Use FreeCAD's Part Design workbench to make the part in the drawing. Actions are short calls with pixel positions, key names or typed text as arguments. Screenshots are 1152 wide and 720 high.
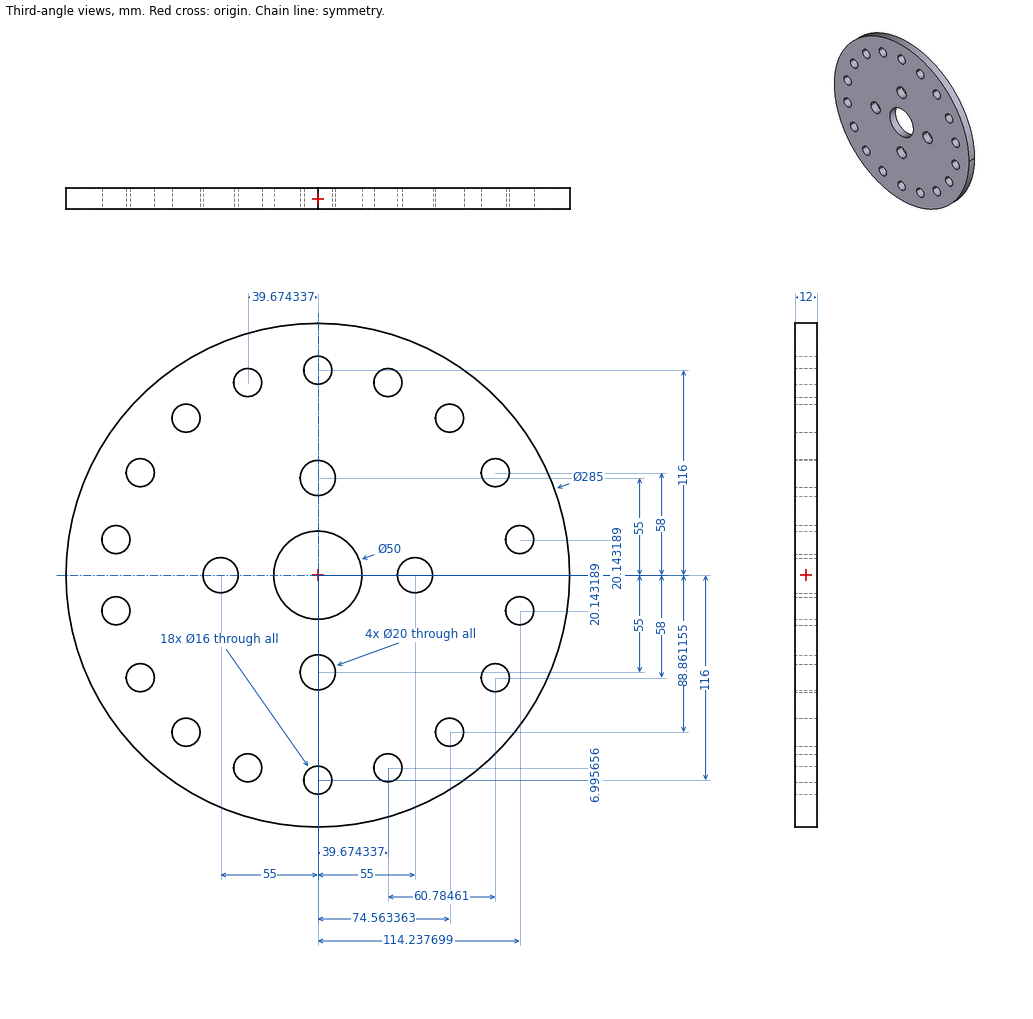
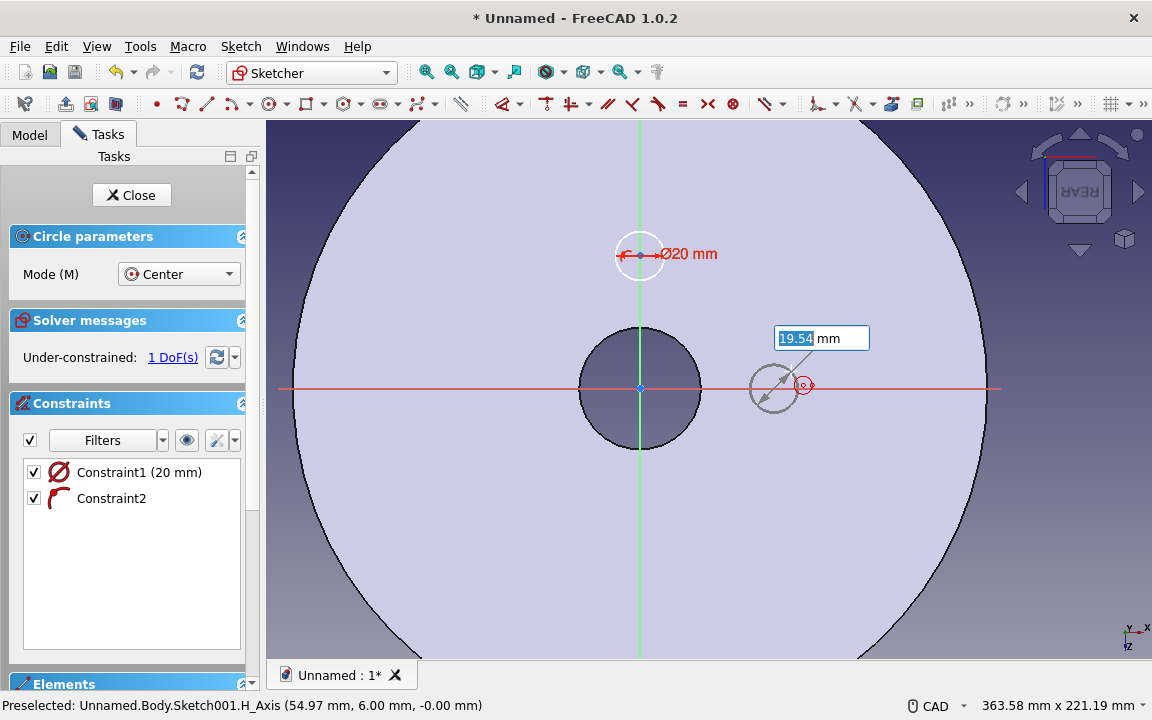
text(20)
key(Return)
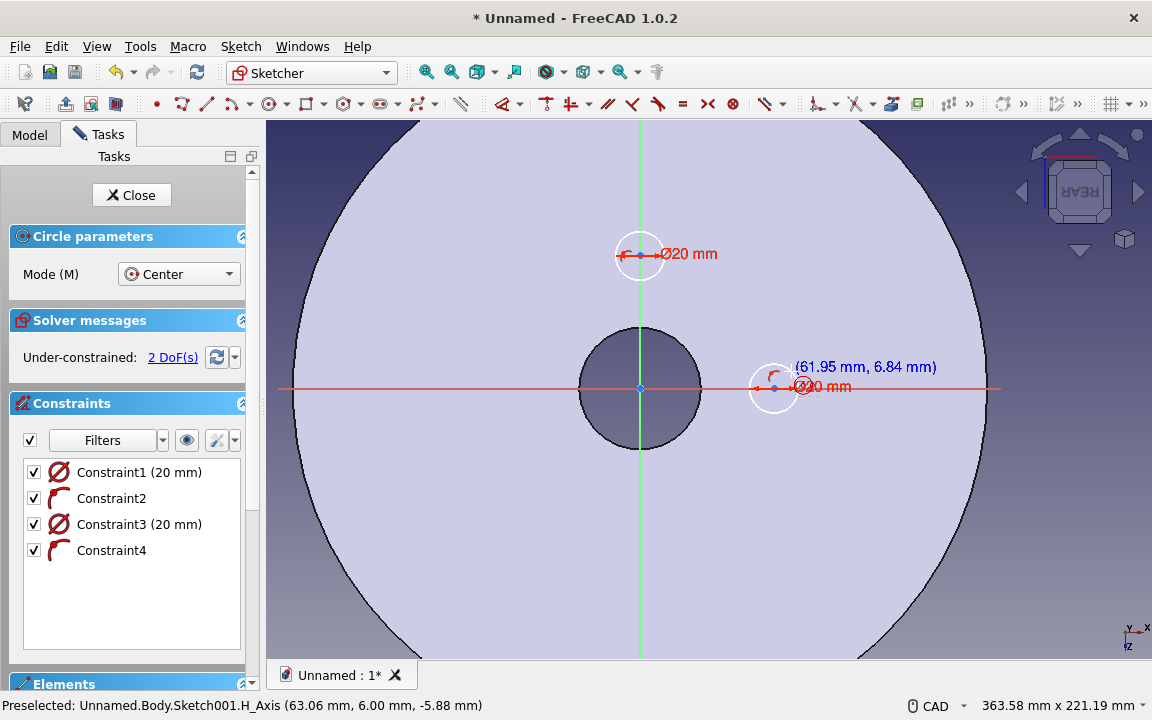
click(640, 523)
move(657, 505)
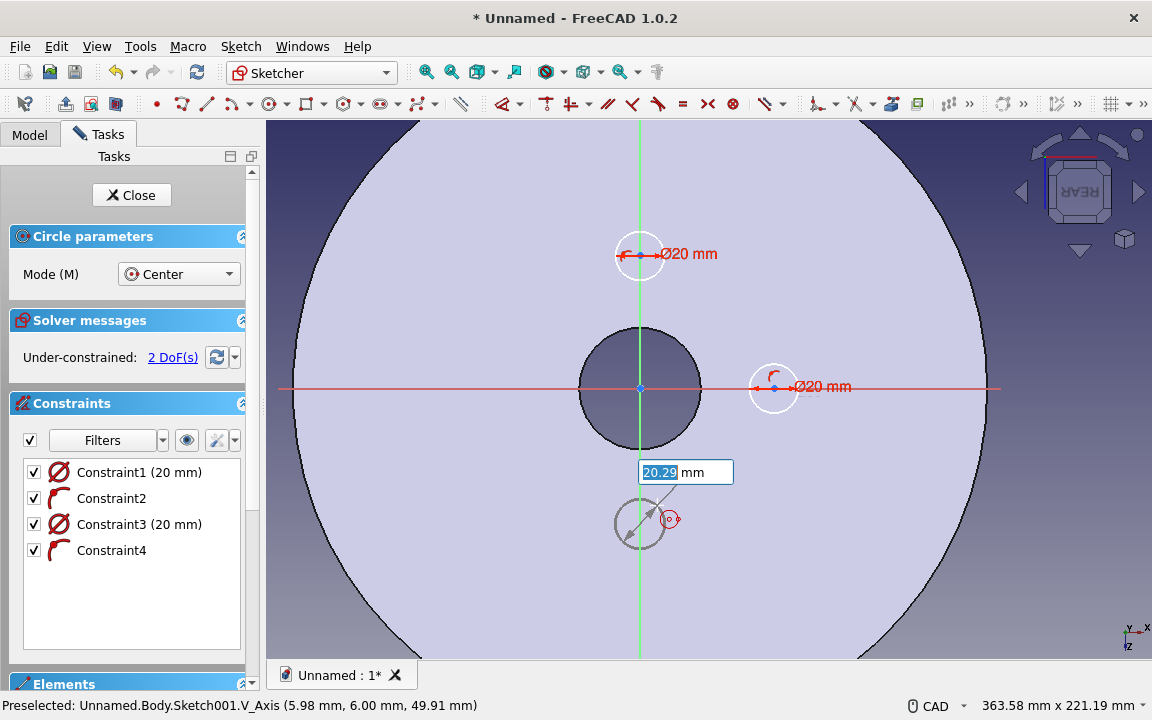
text(20)
key(Return)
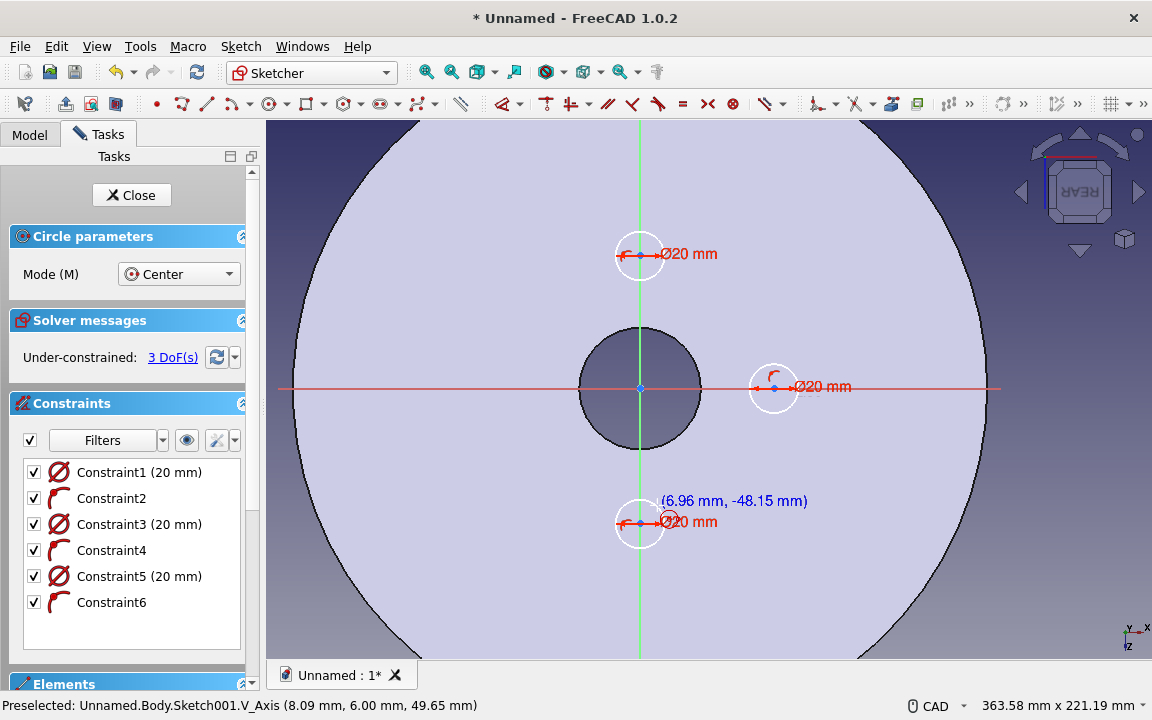
click(506, 389)
move(523, 371)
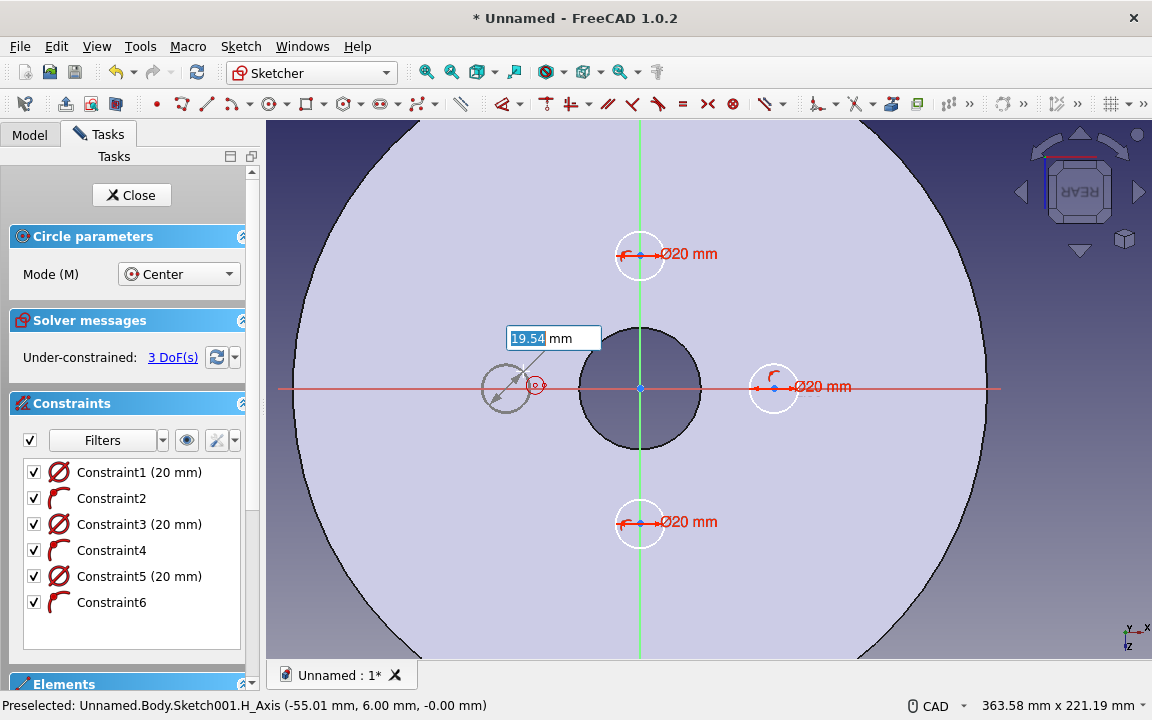
text(20)
key(Return)
key(Escape)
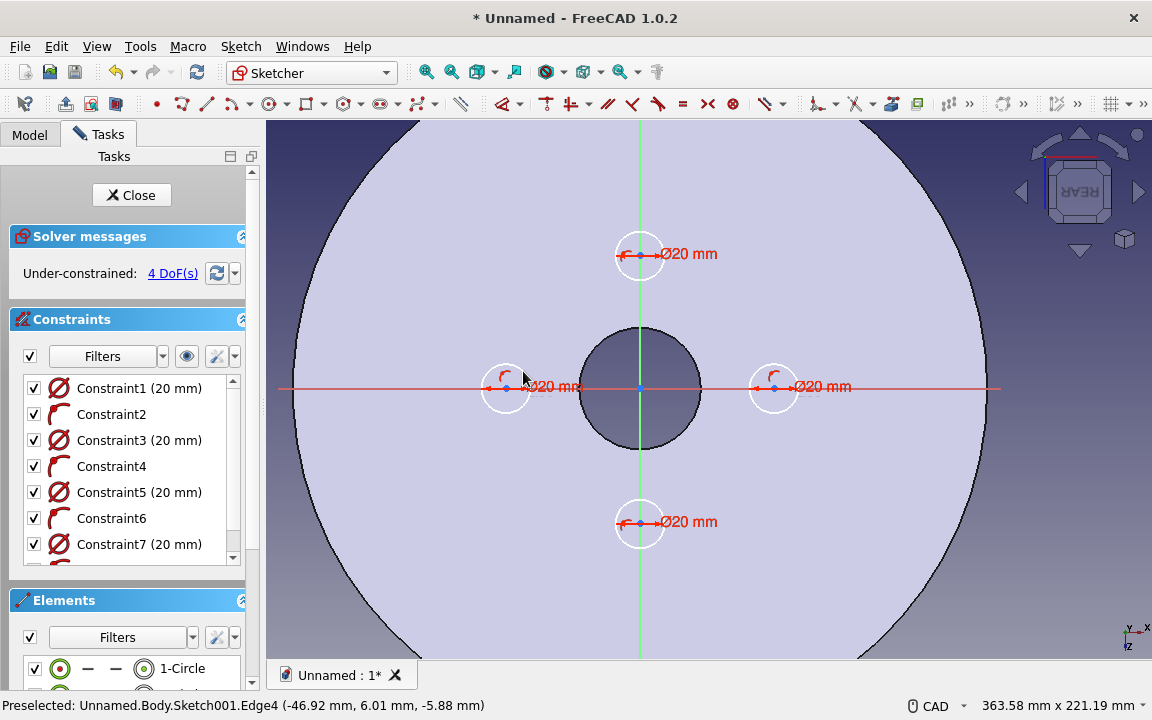
click(502, 104)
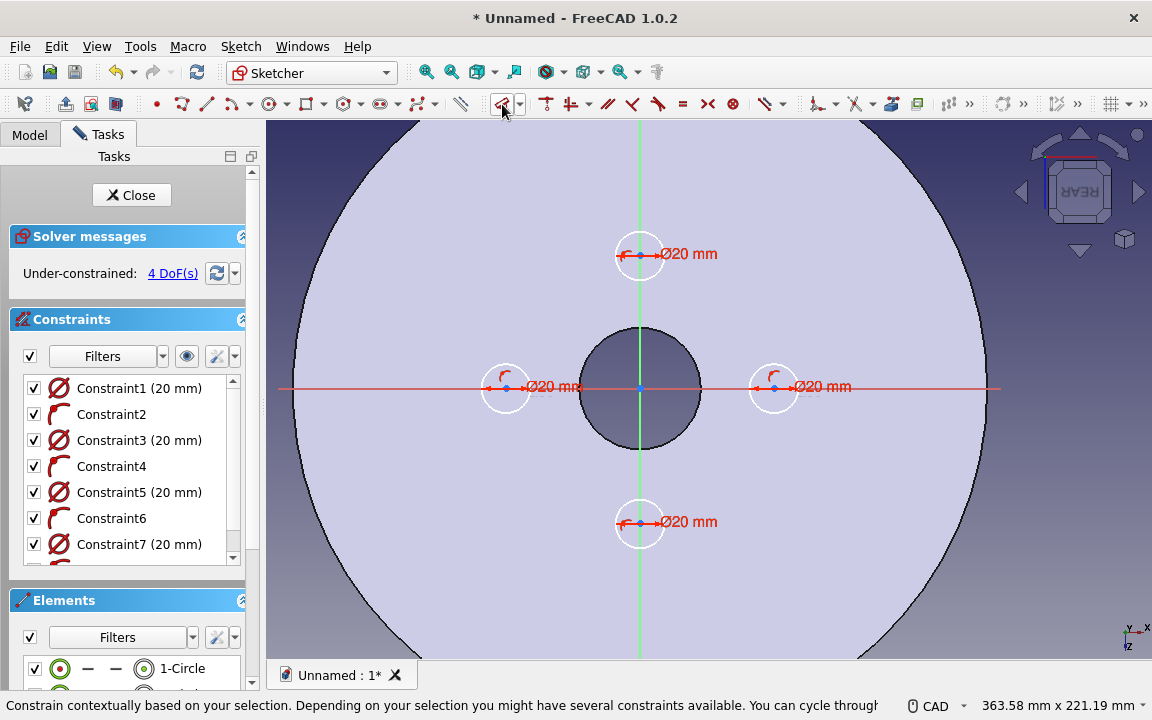
click(640, 256)
click(674, 322)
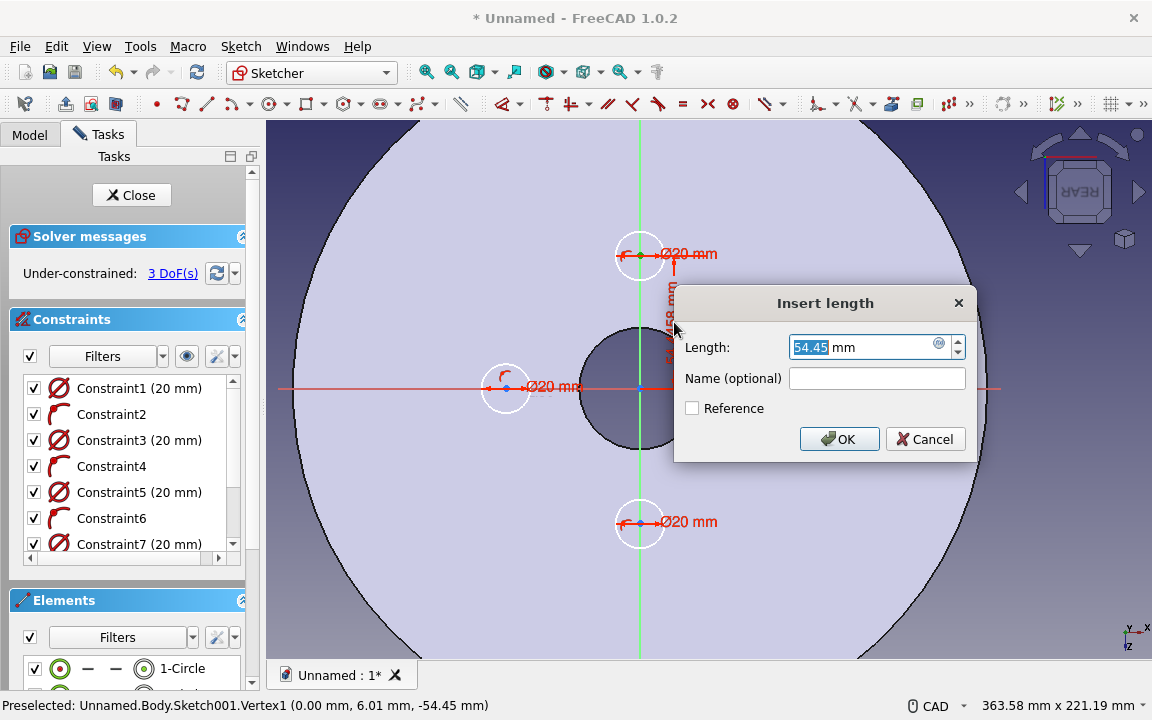
text(55)
key(Return)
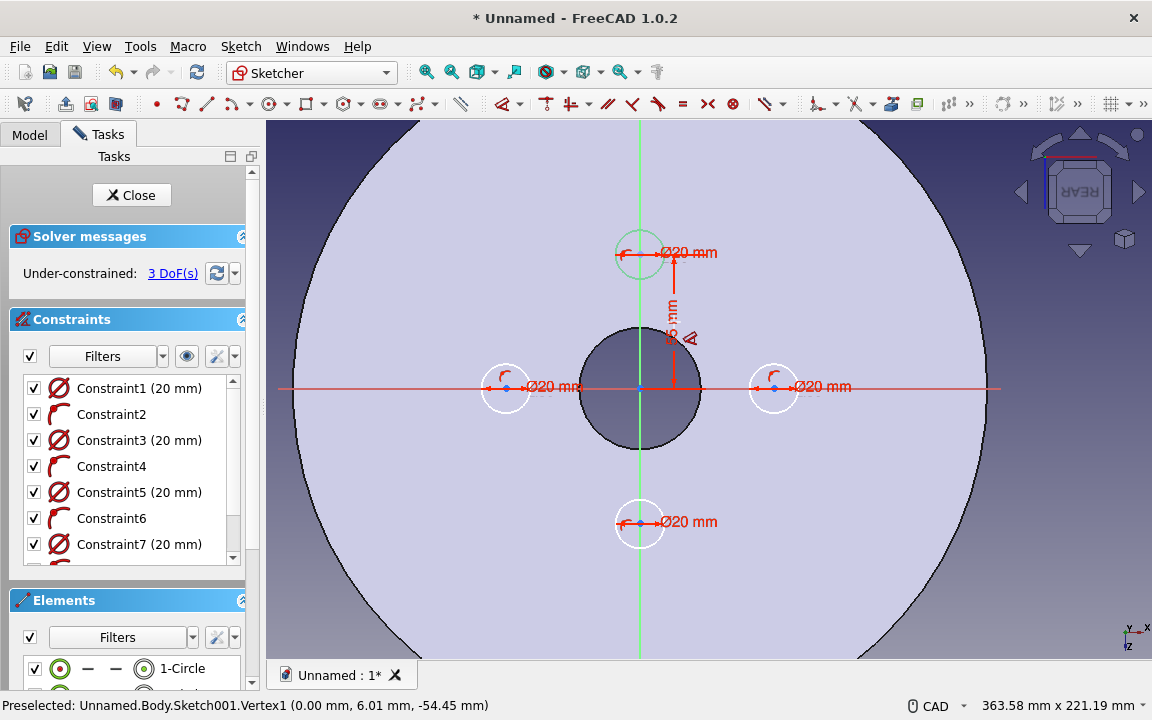
click(774, 389)
click(707, 423)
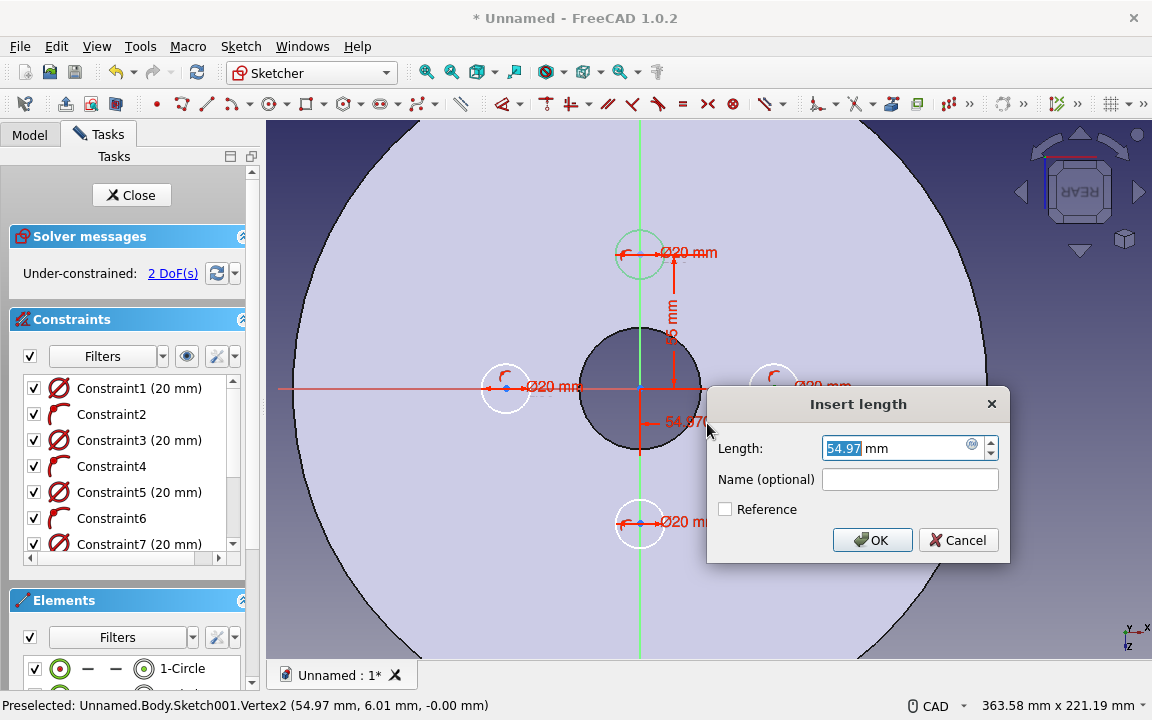
text(55)
key(Return)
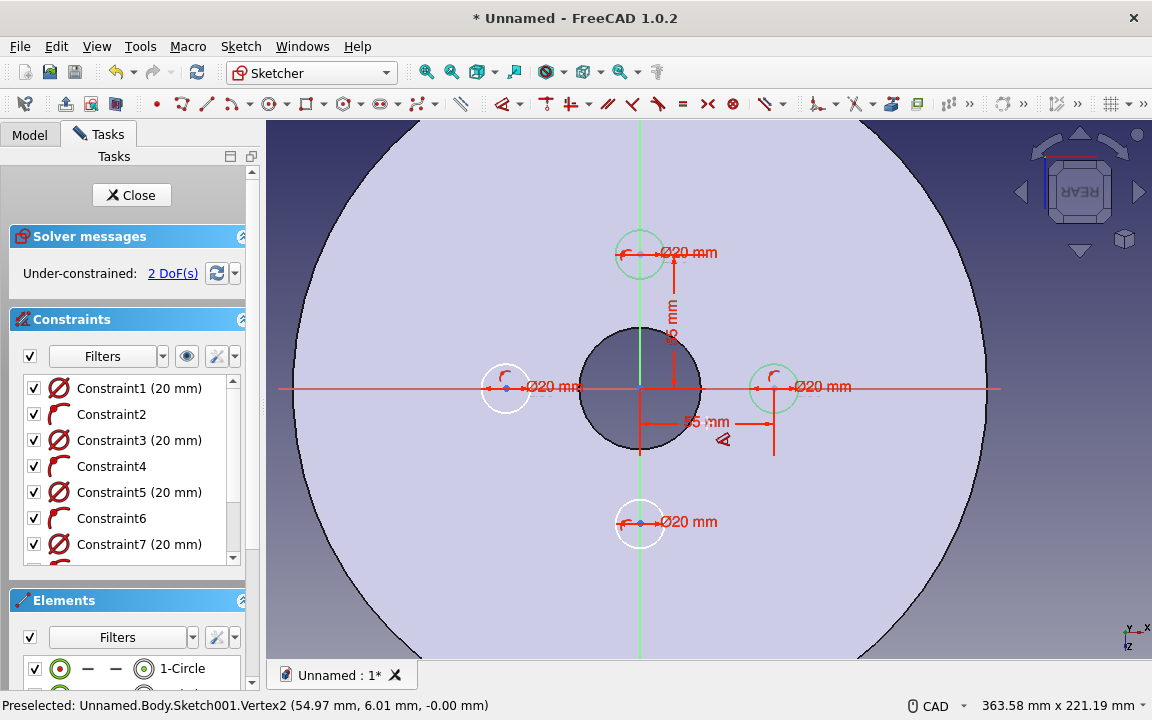
click(640, 524)
click(674, 456)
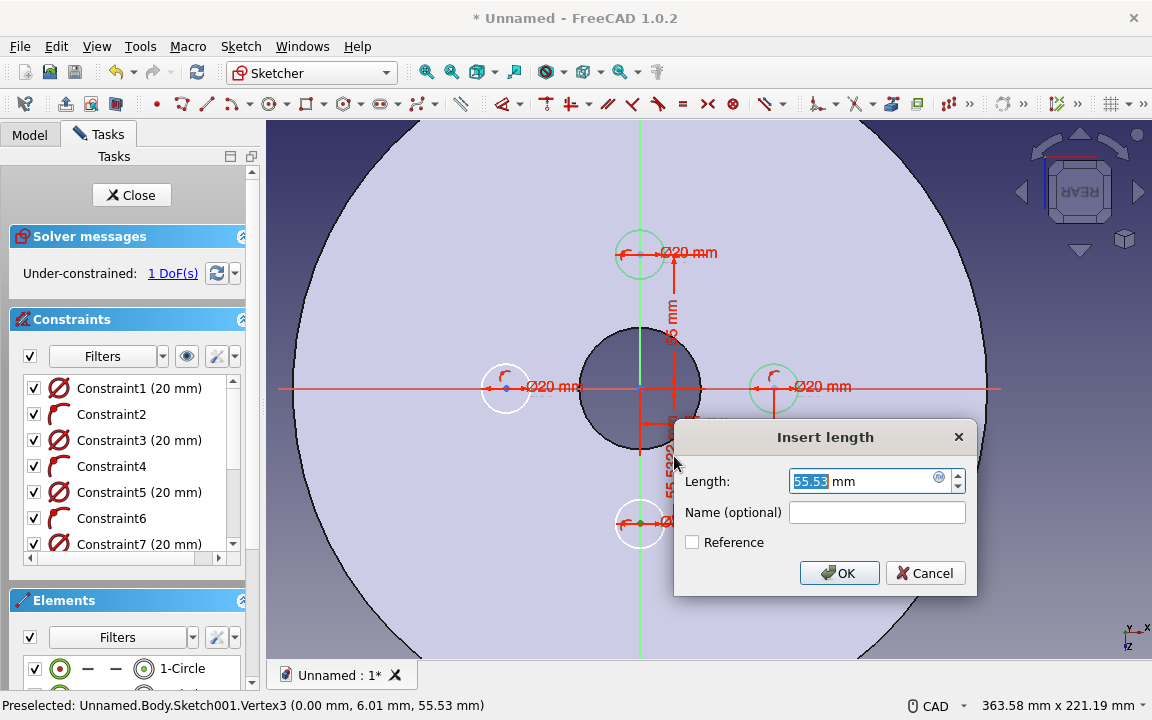
text(55)
key(Return)